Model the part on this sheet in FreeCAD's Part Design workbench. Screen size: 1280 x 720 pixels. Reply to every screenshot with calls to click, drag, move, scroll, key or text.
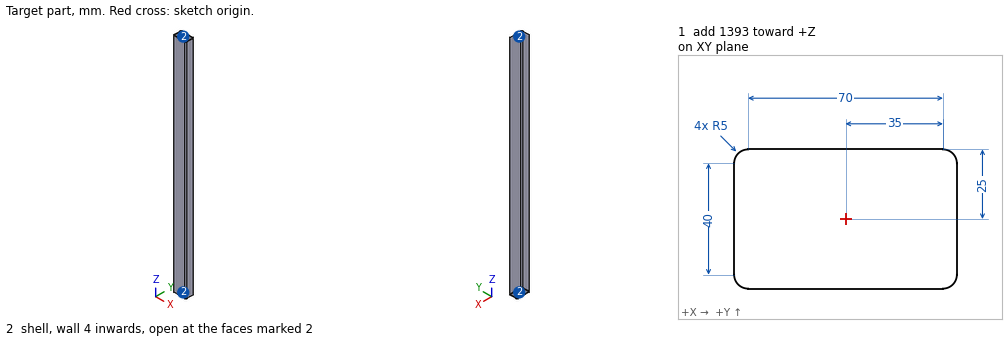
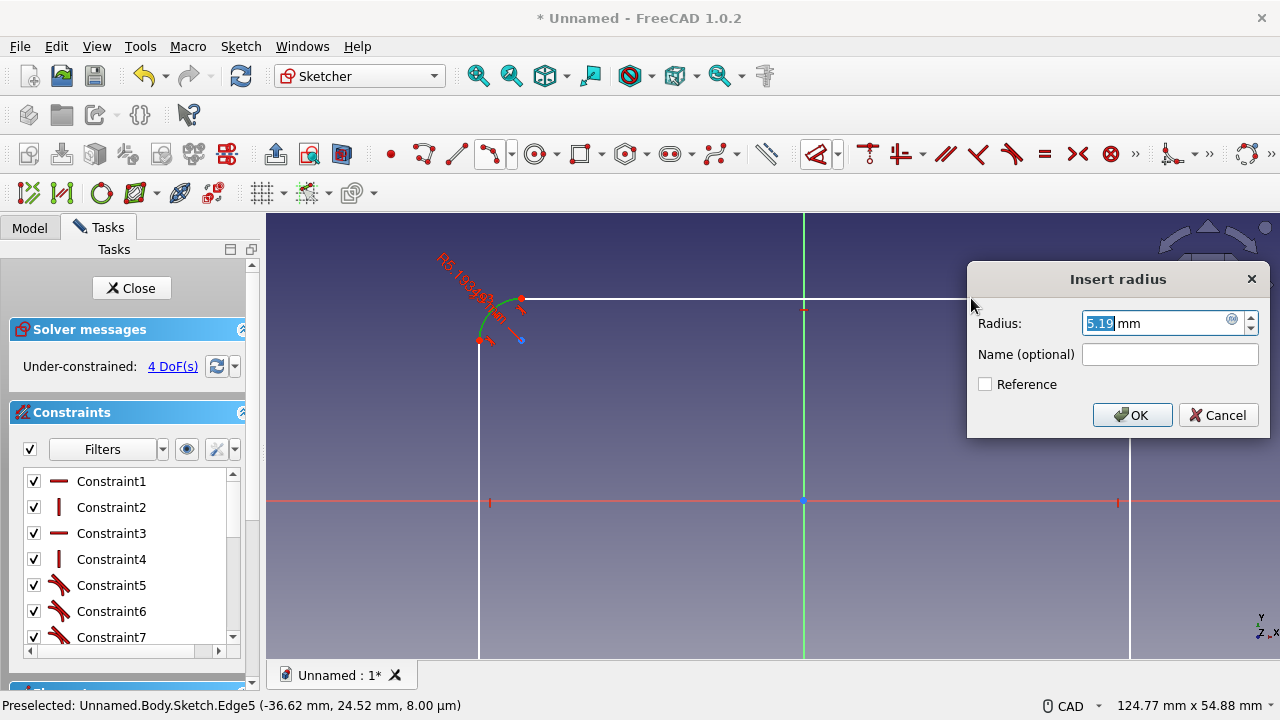
text(5)
key(Return)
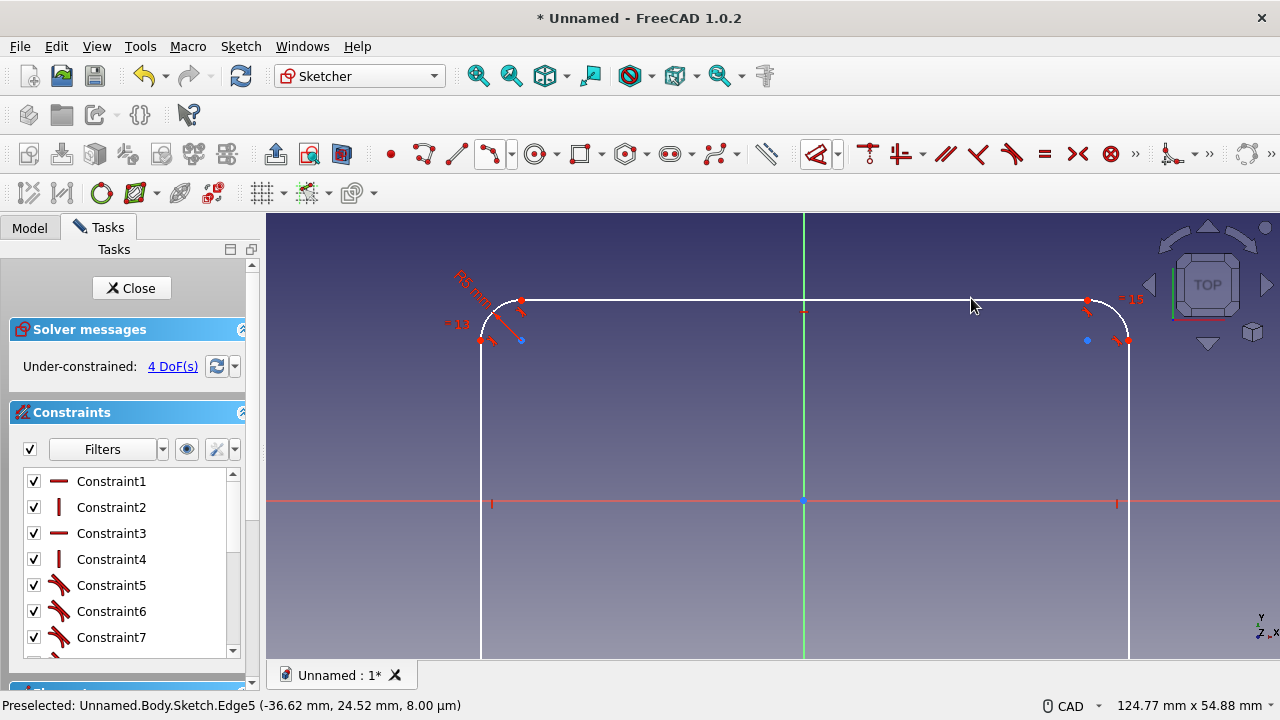
click(918, 300)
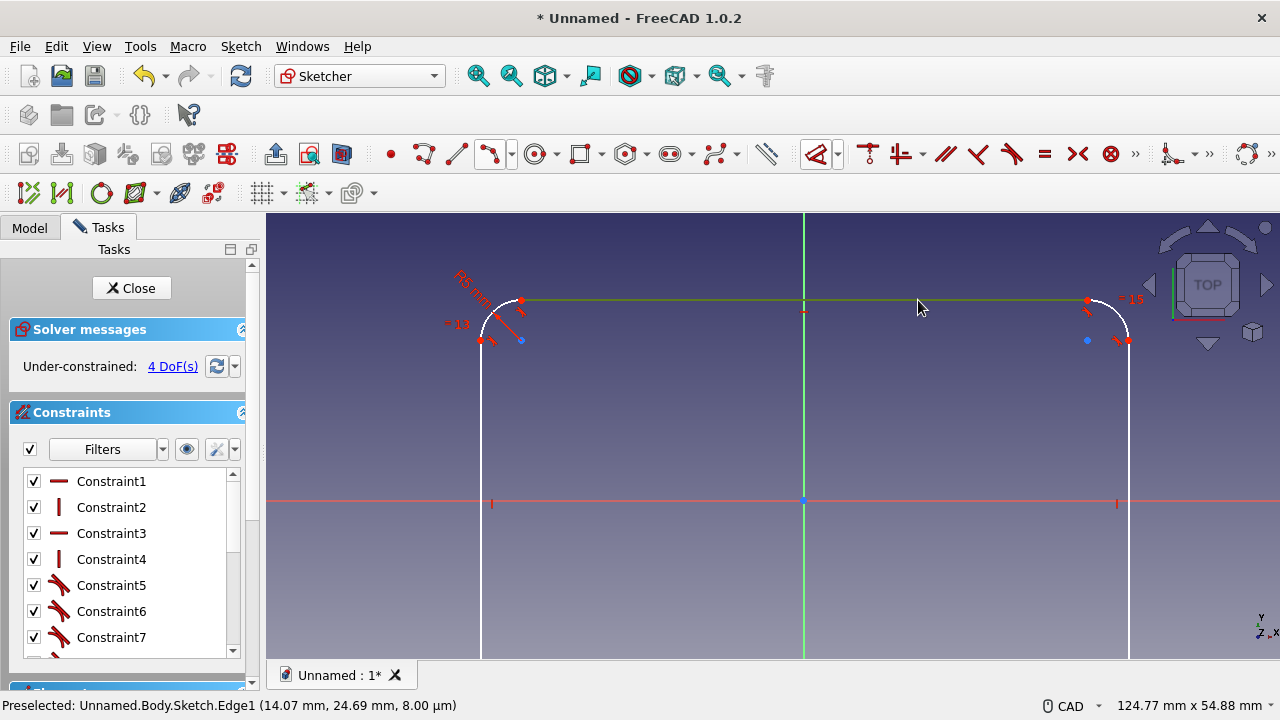
click(838, 154)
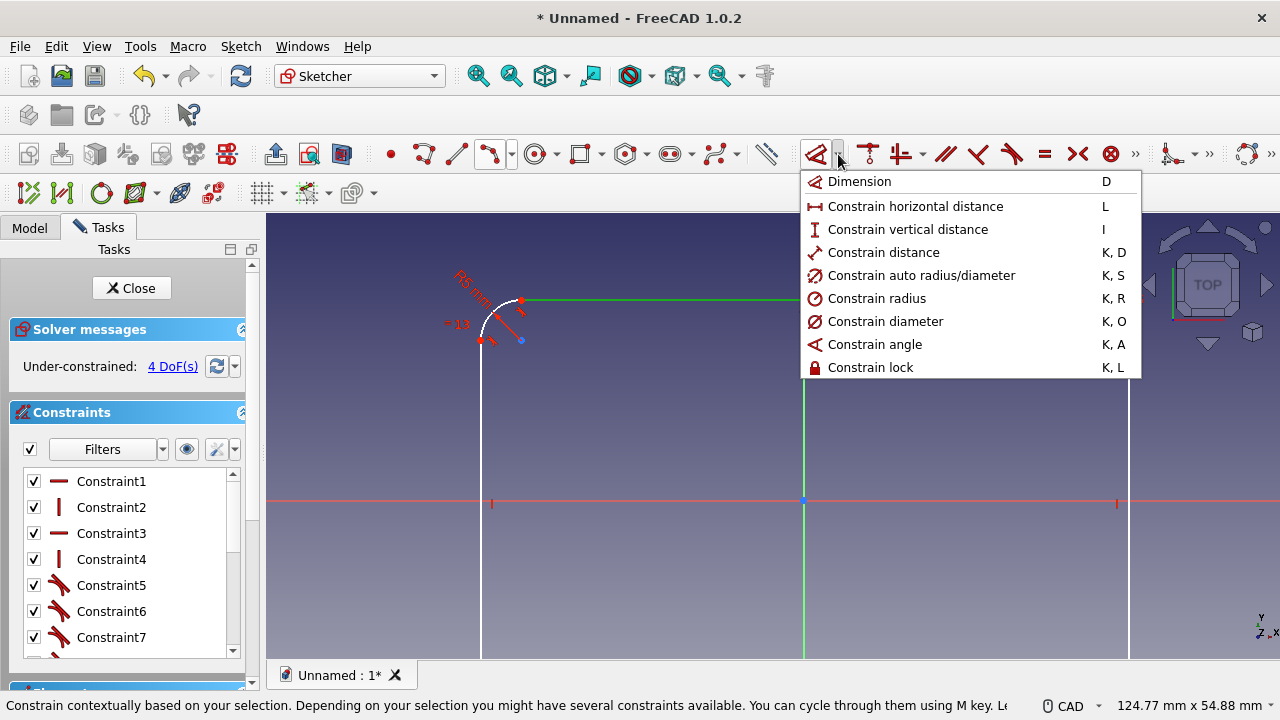
click(971, 206)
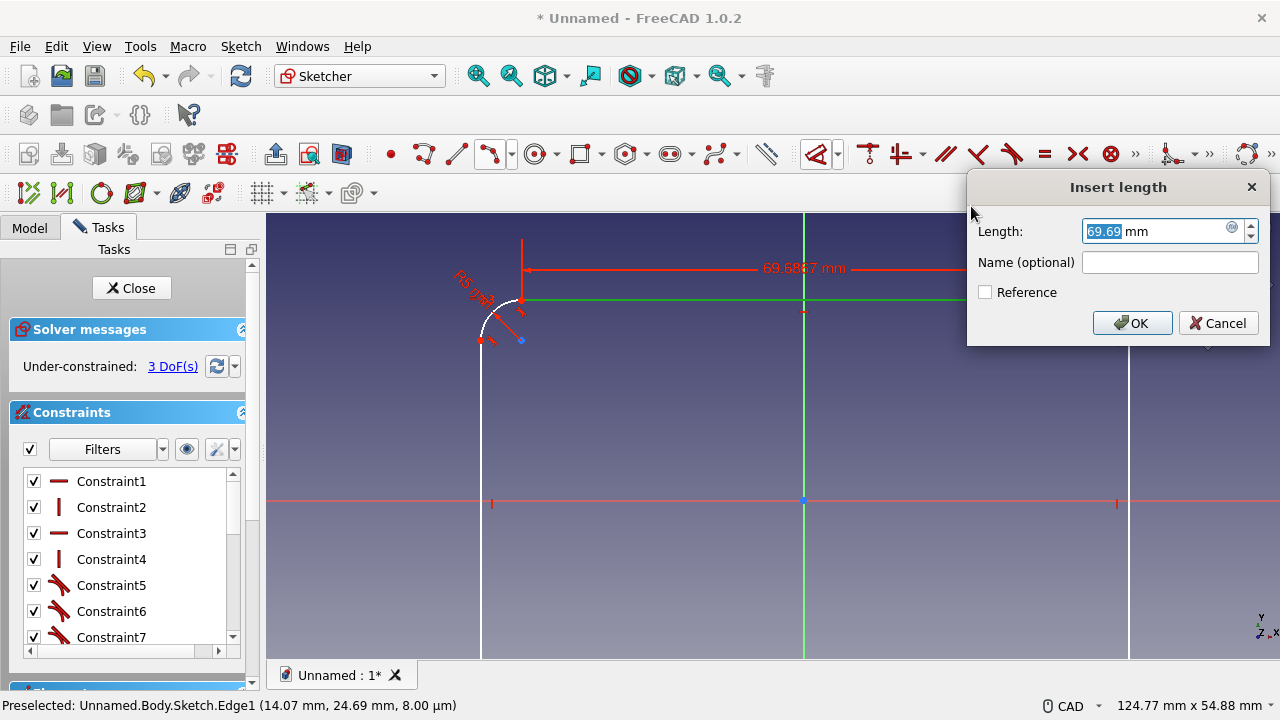
text(70)
key(Return)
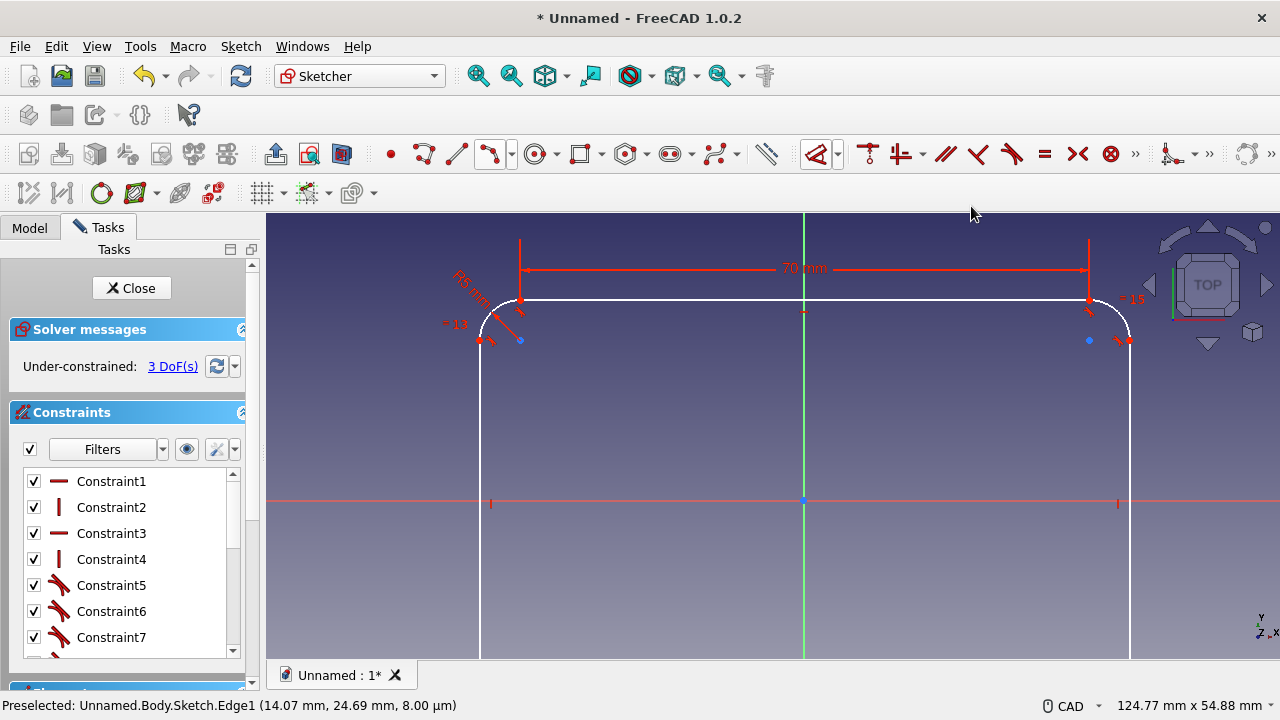
click(480, 439)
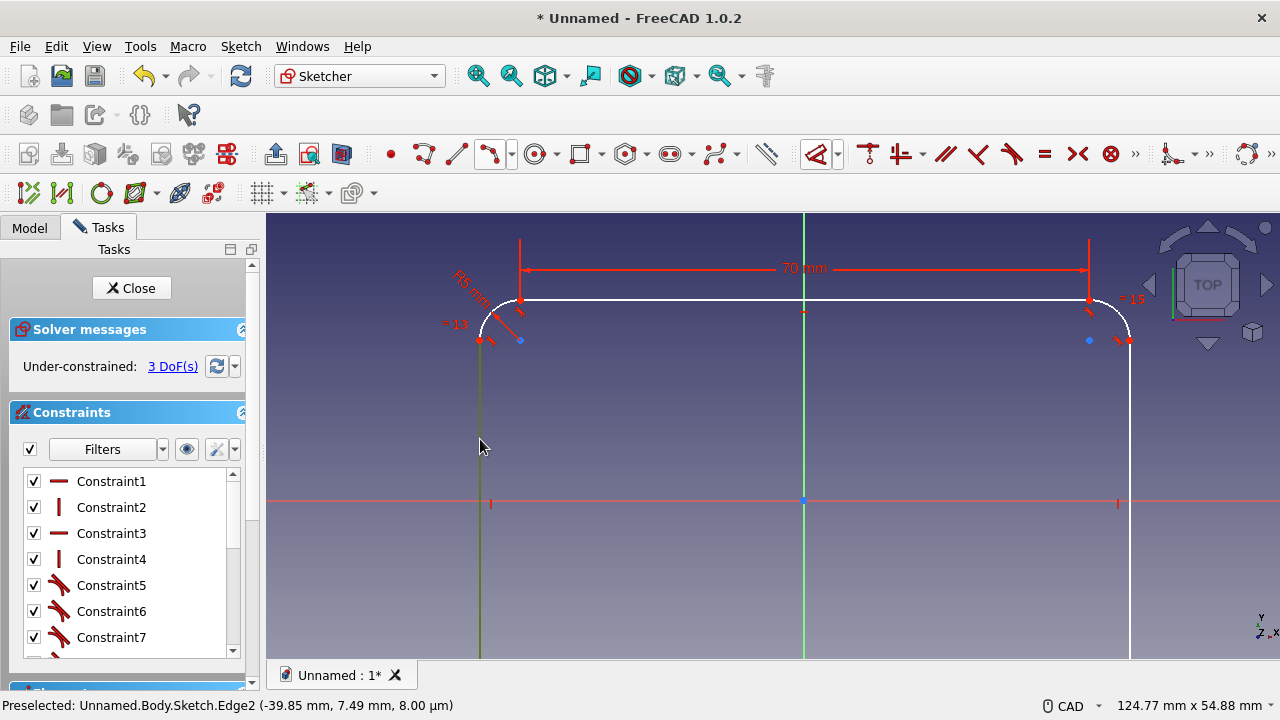
key(i)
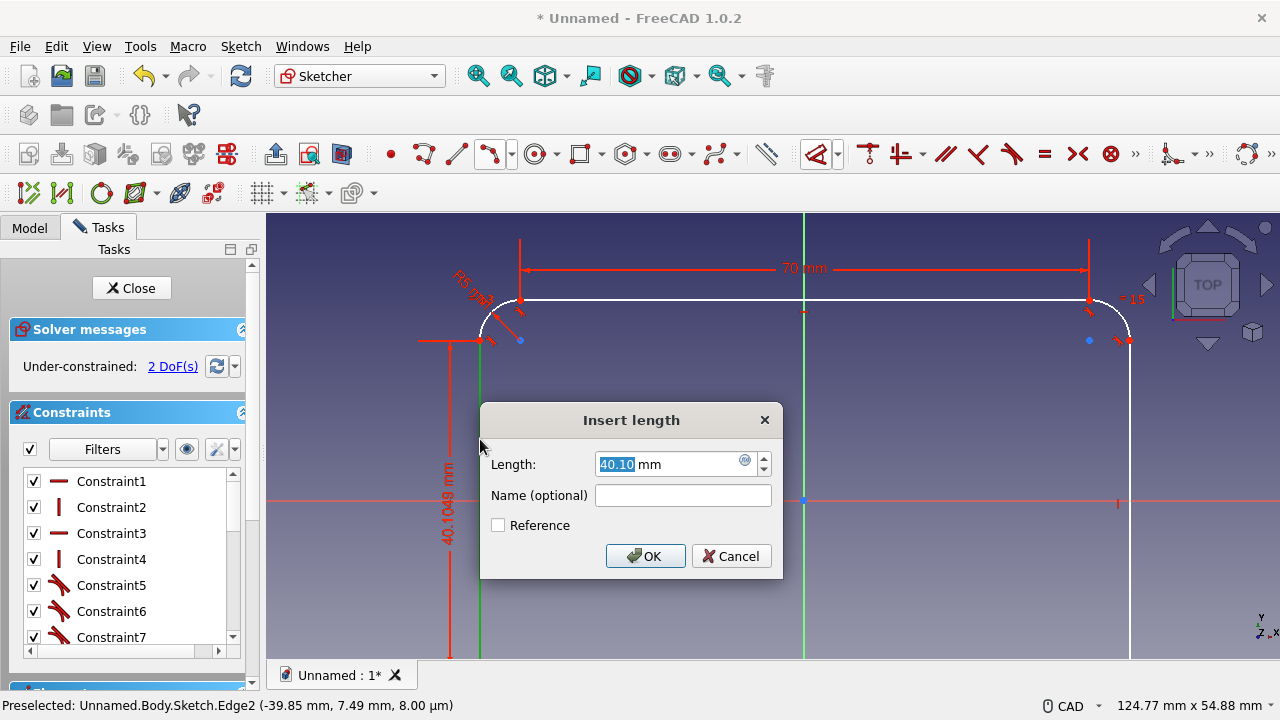
text(40)
key(Return)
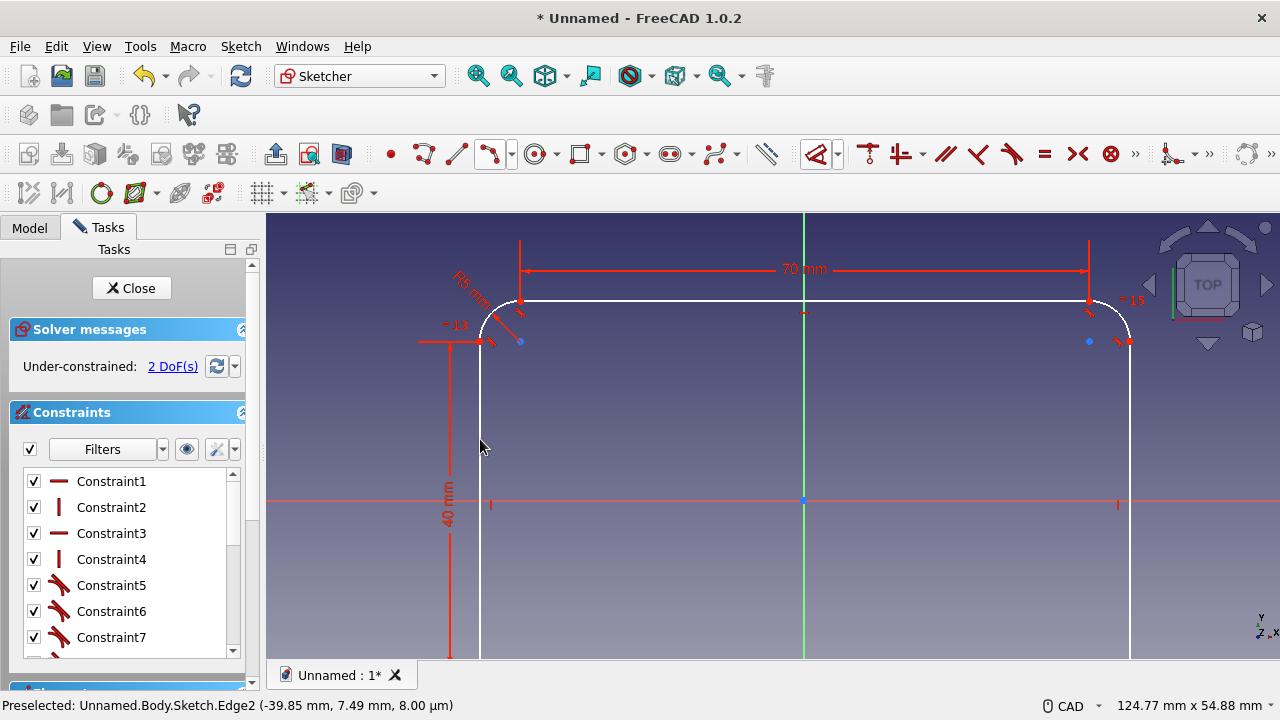
click(1089, 301)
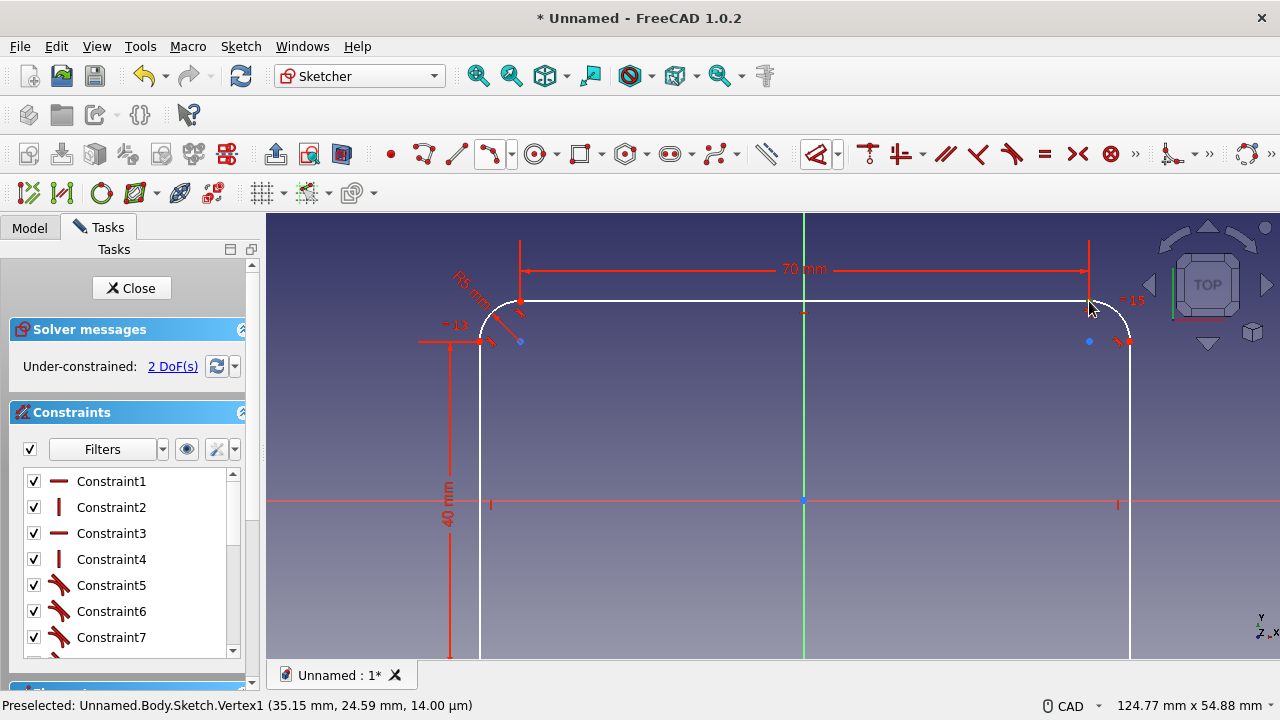
click(838, 154)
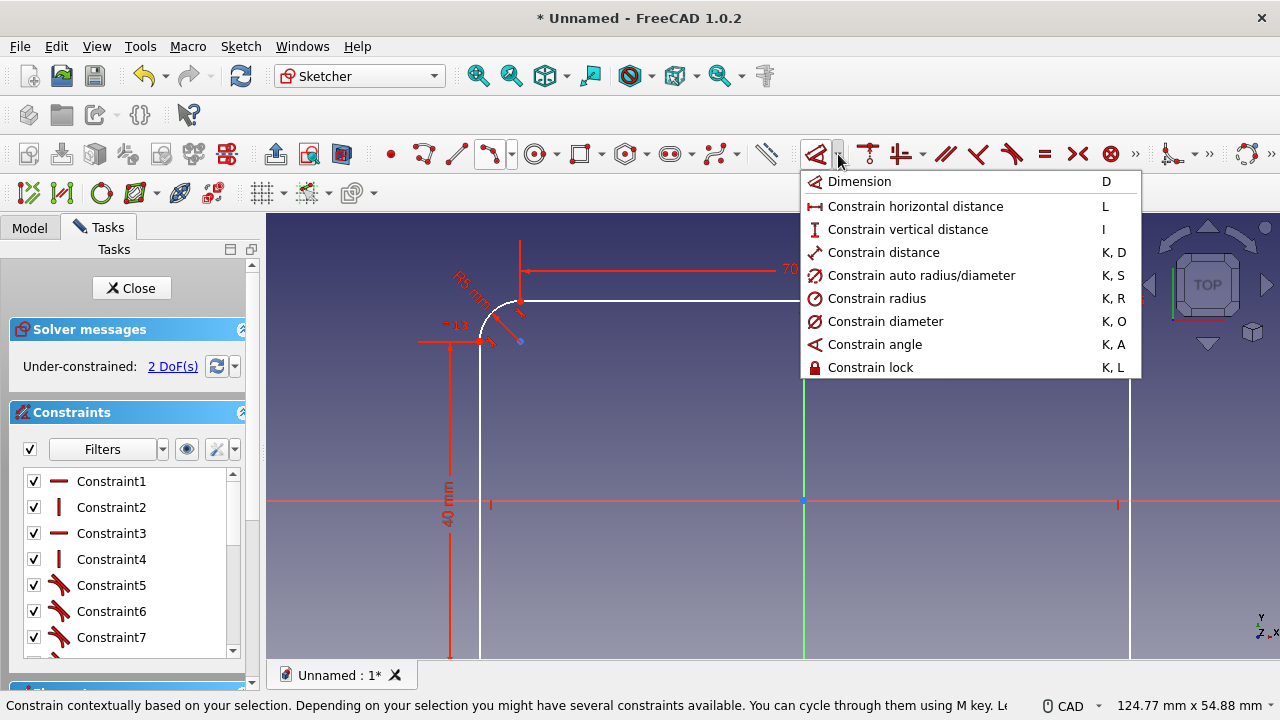
click(971, 206)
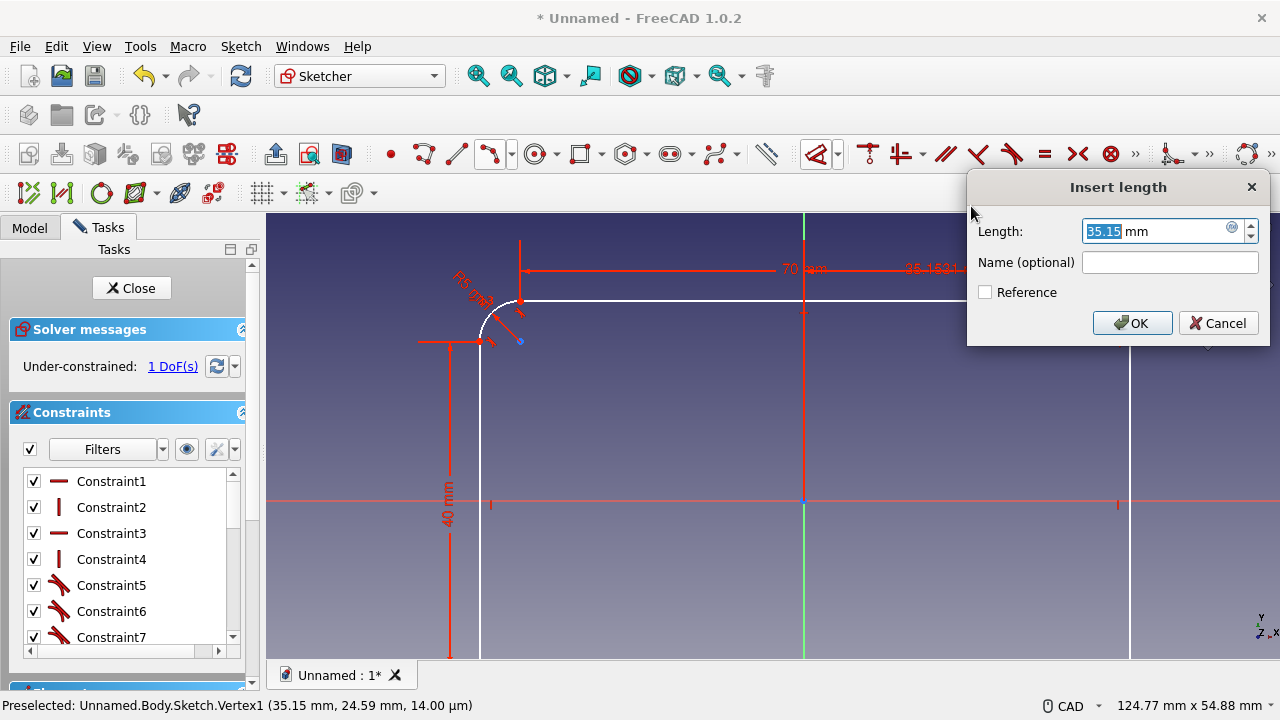
text(35)
key(Return)